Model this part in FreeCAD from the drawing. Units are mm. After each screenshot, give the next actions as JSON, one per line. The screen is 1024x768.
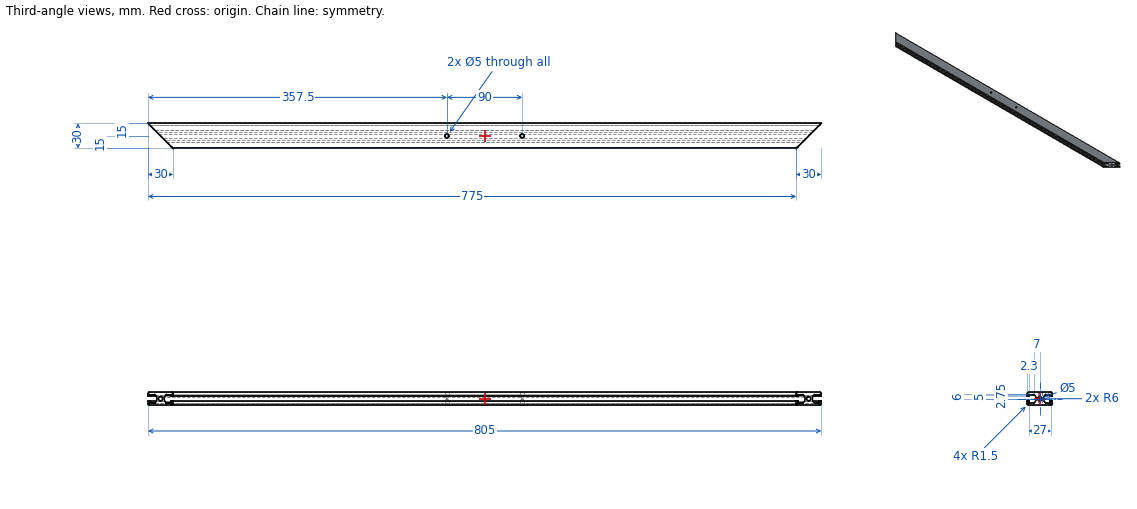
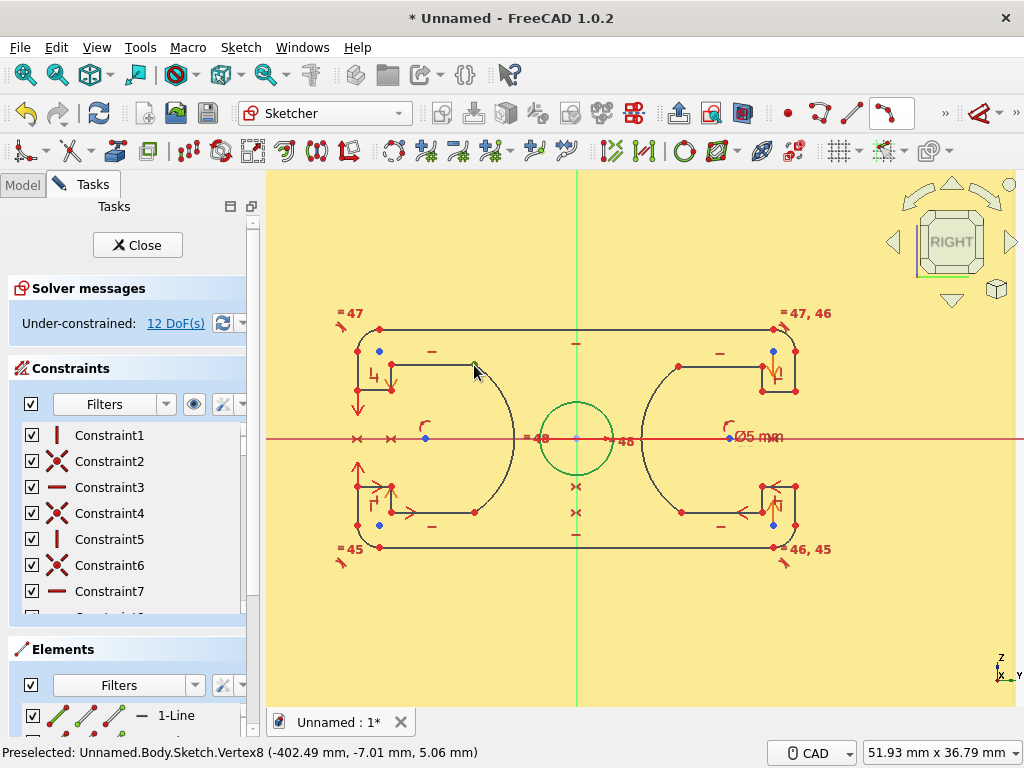
{"action": "left_click", "coordinate": [678, 367]}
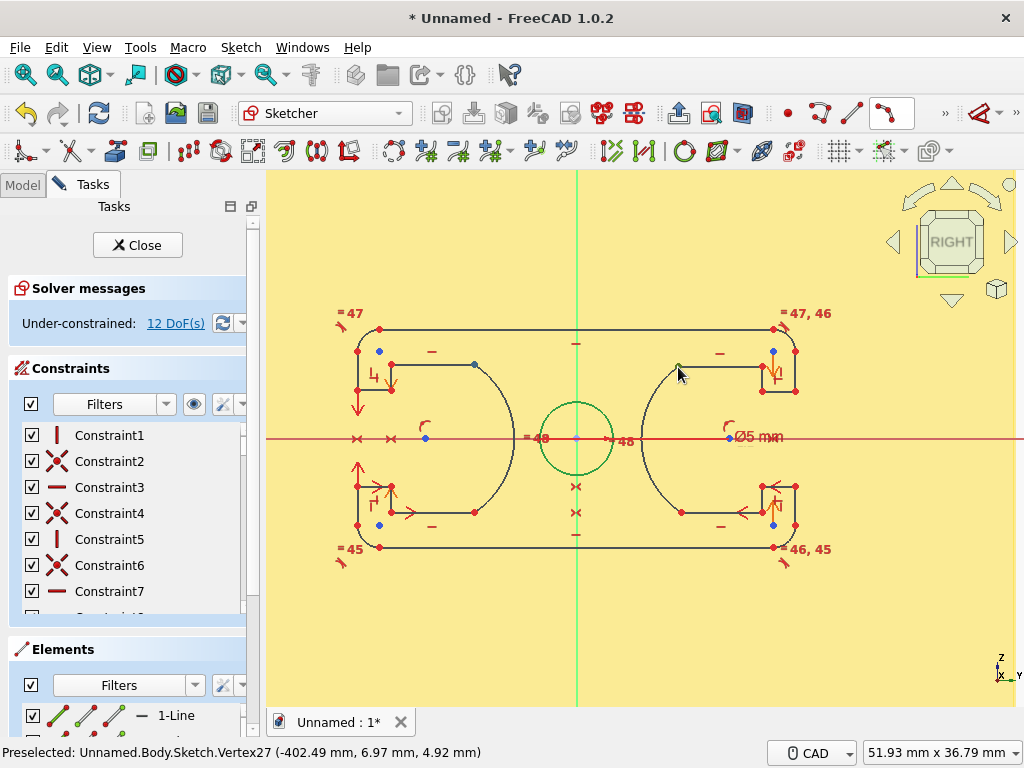
{"action": "left_click", "coordinate": [577, 645]}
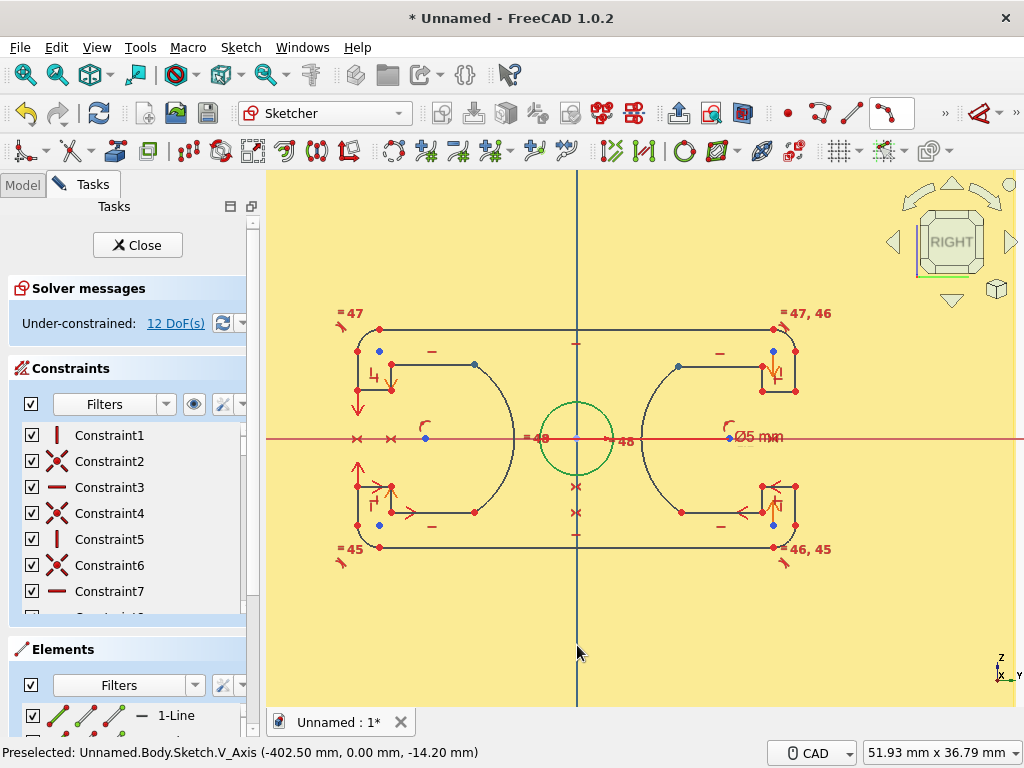
{"action": "key", "text": "s"}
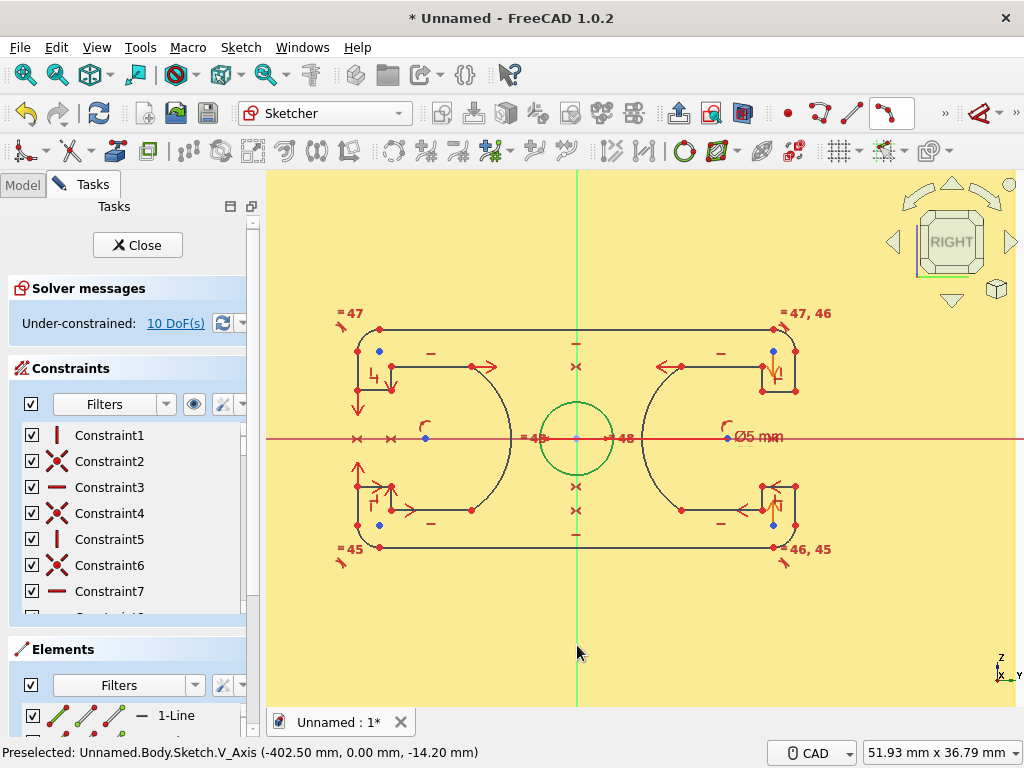
{"action": "left_click", "coordinate": [391, 390]}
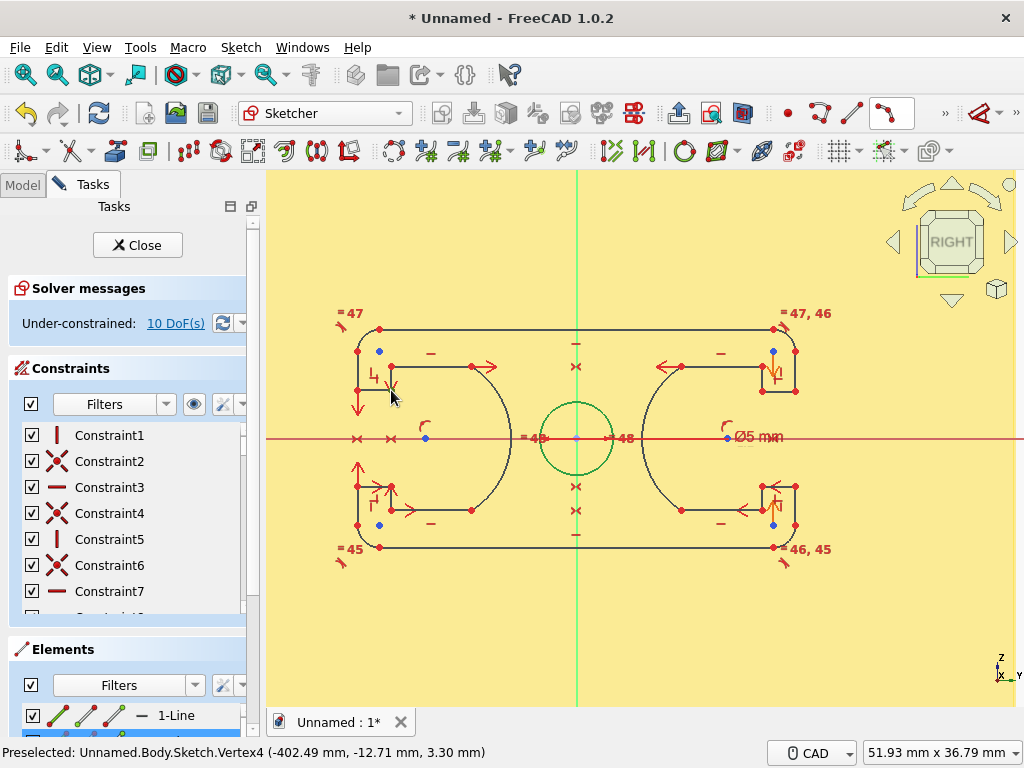
{"action": "left_click", "coordinate": [762, 392]}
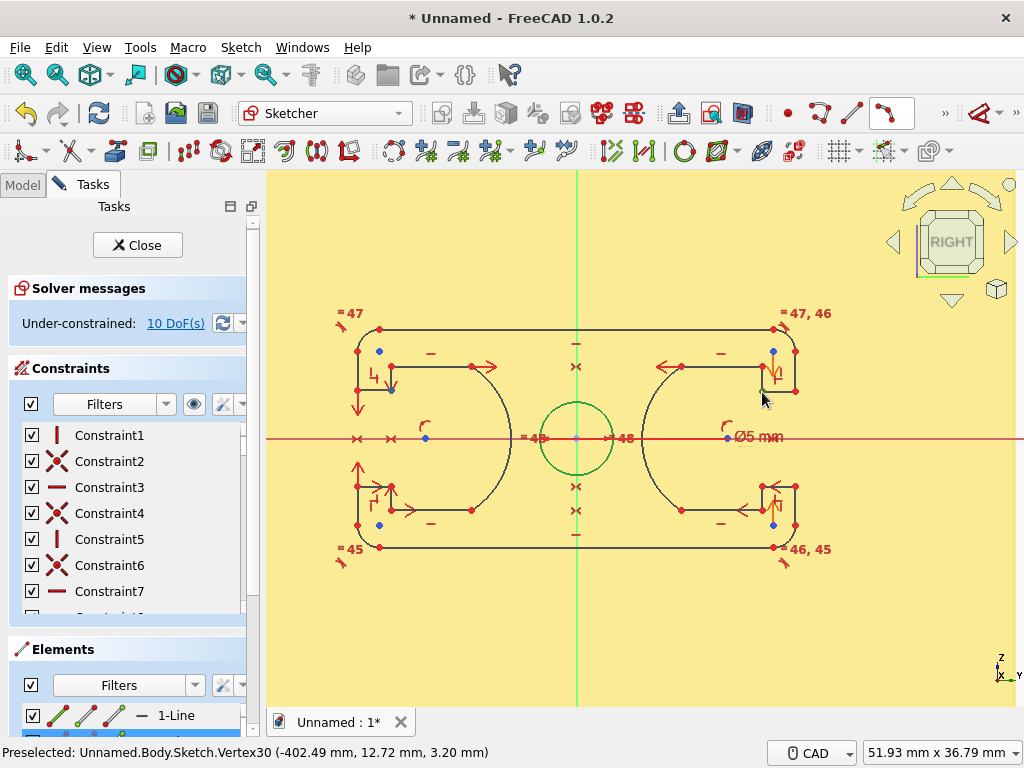
{"action": "left_click", "coordinate": [577, 645]}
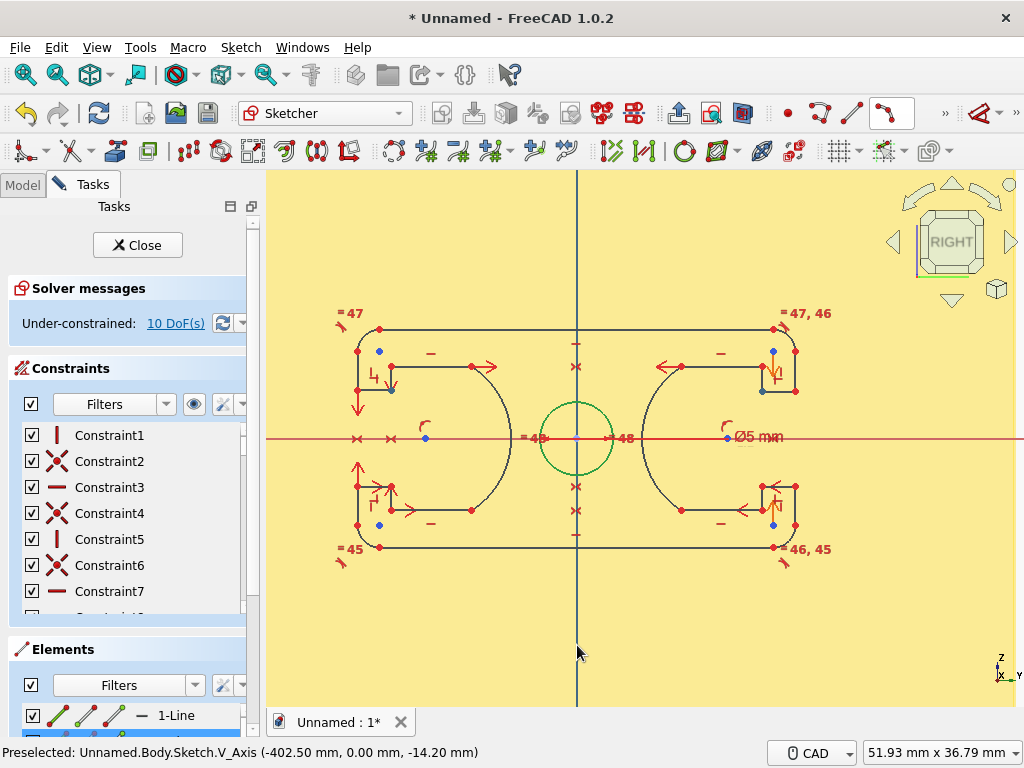
{"action": "key", "text": "s"}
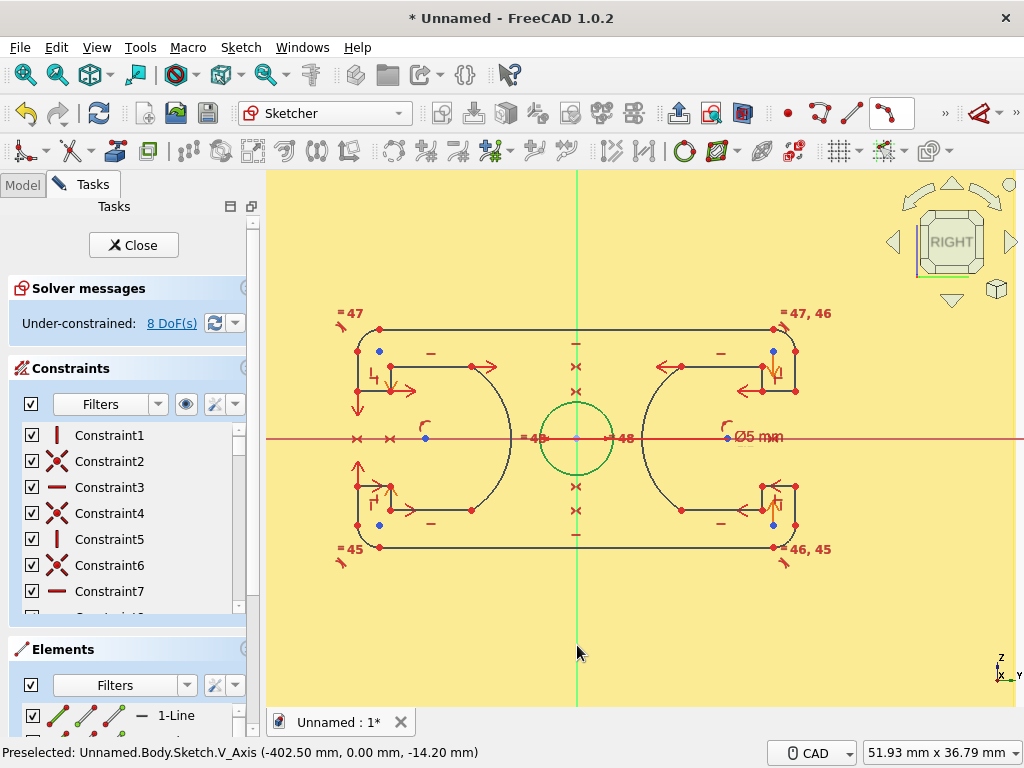
{"action": "left_click", "coordinate": [504, 472]}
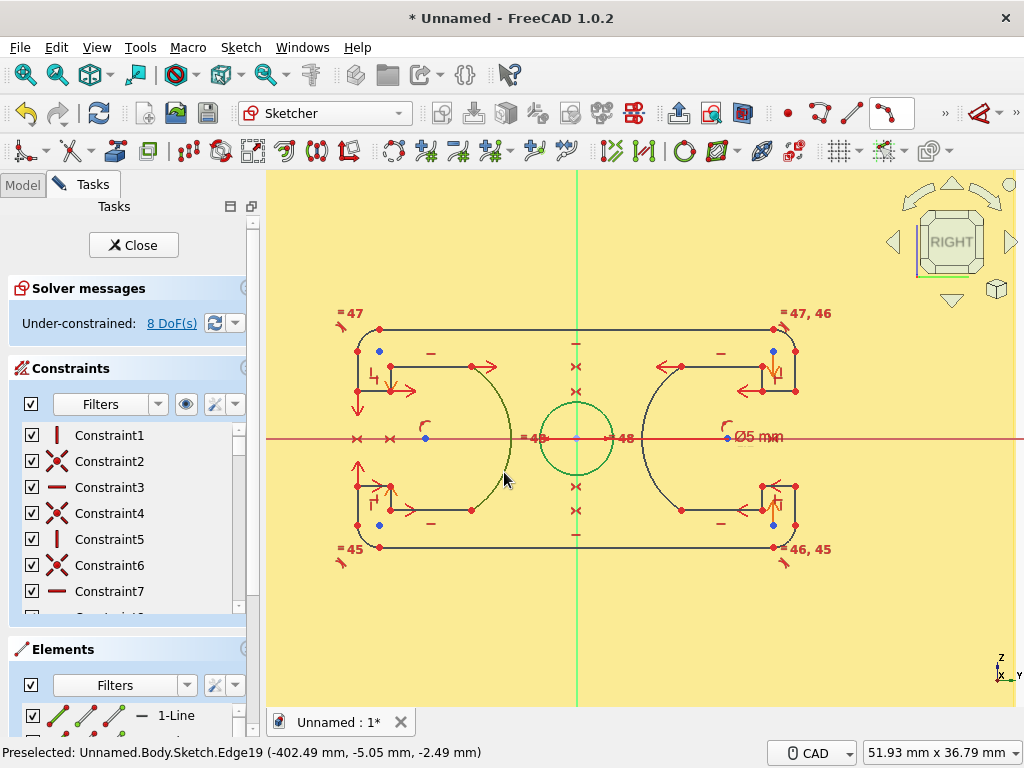
{"action": "key", "text": "k r"}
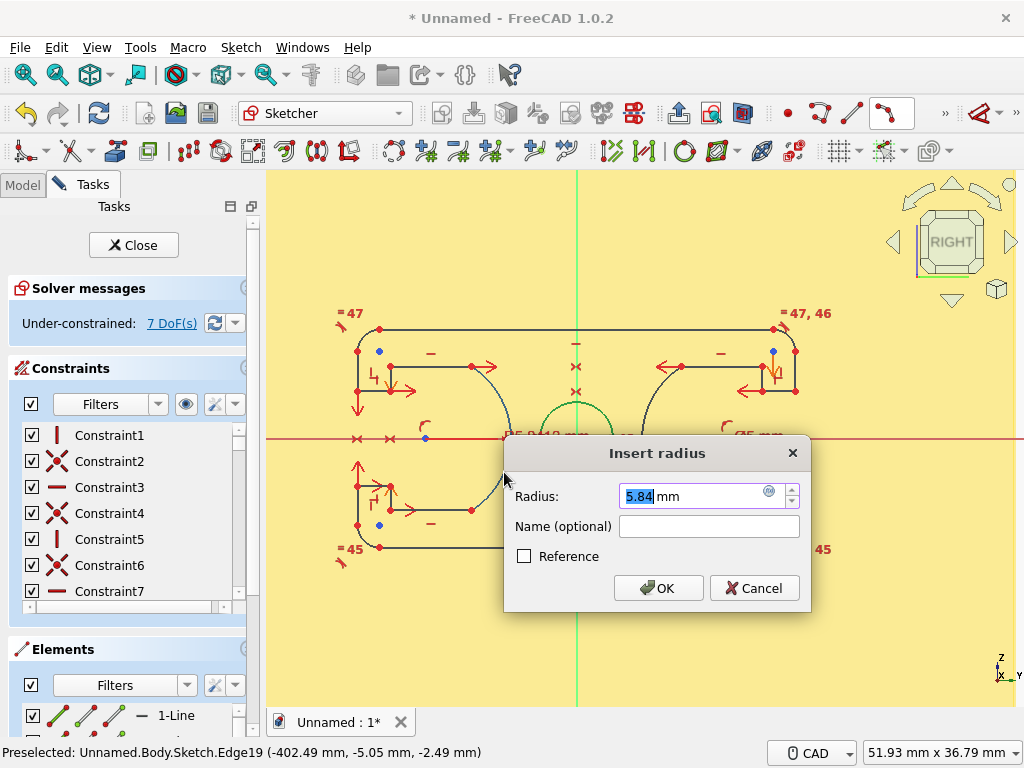
{"action": "type", "text": "6"}
{"action": "key", "text": "Return"}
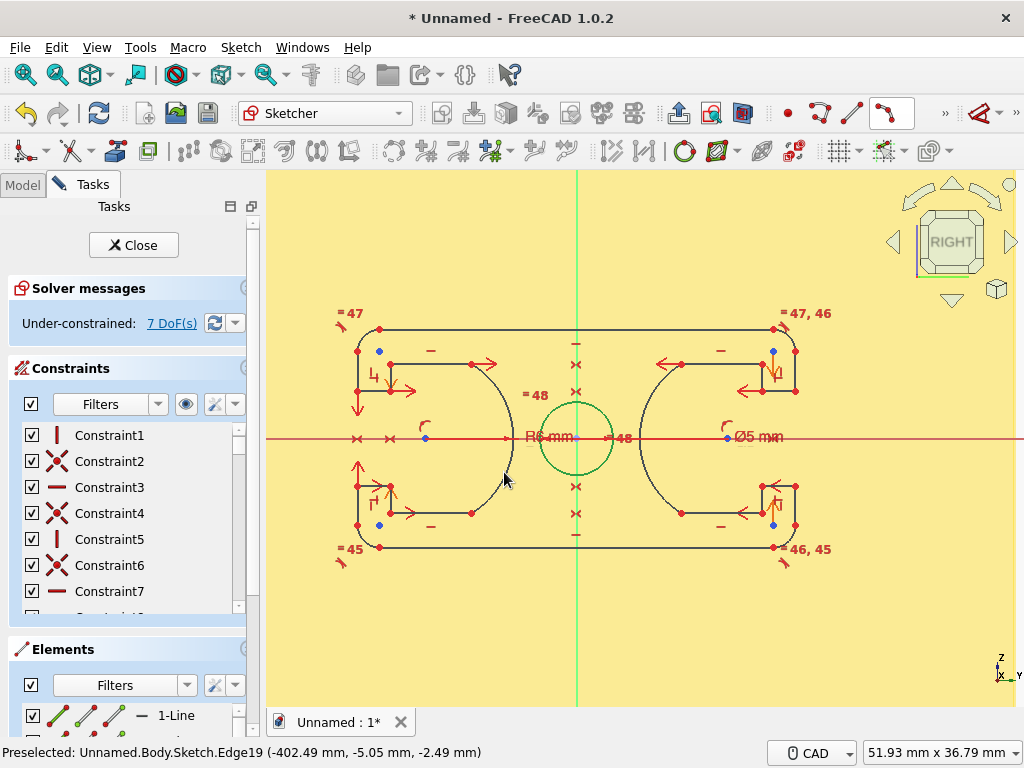
{"action": "scroll", "coordinate": [360, 536], "scroll_direction": "up", "scroll_amount": 3}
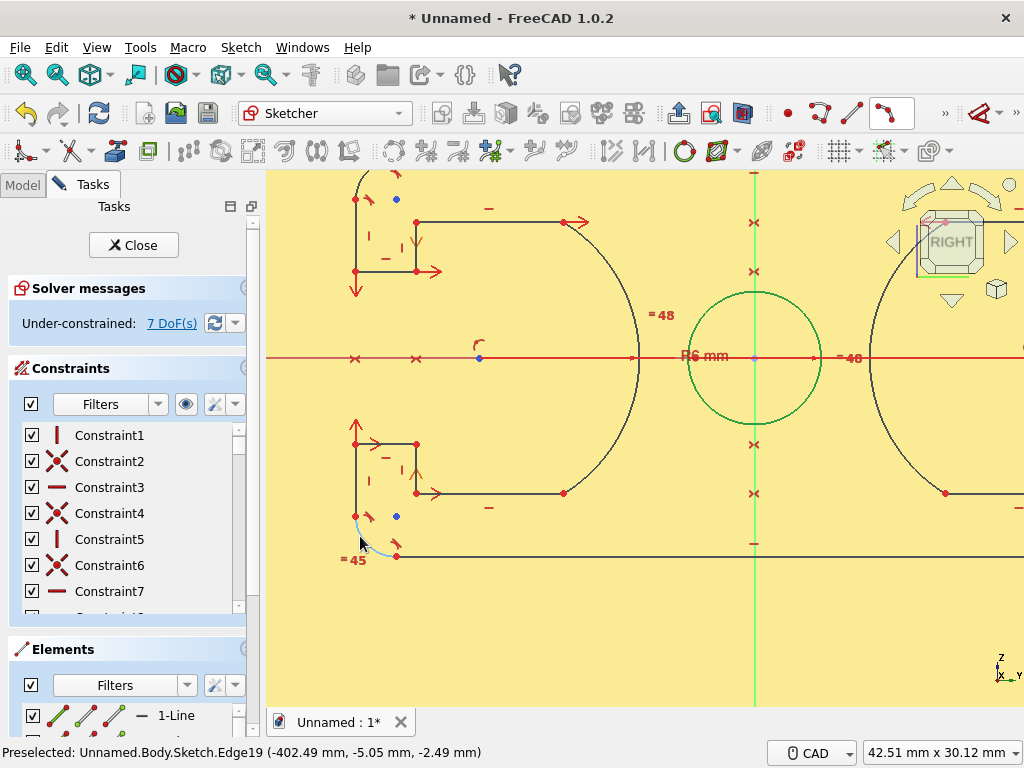
{"action": "left_click", "coordinate": [360, 535]}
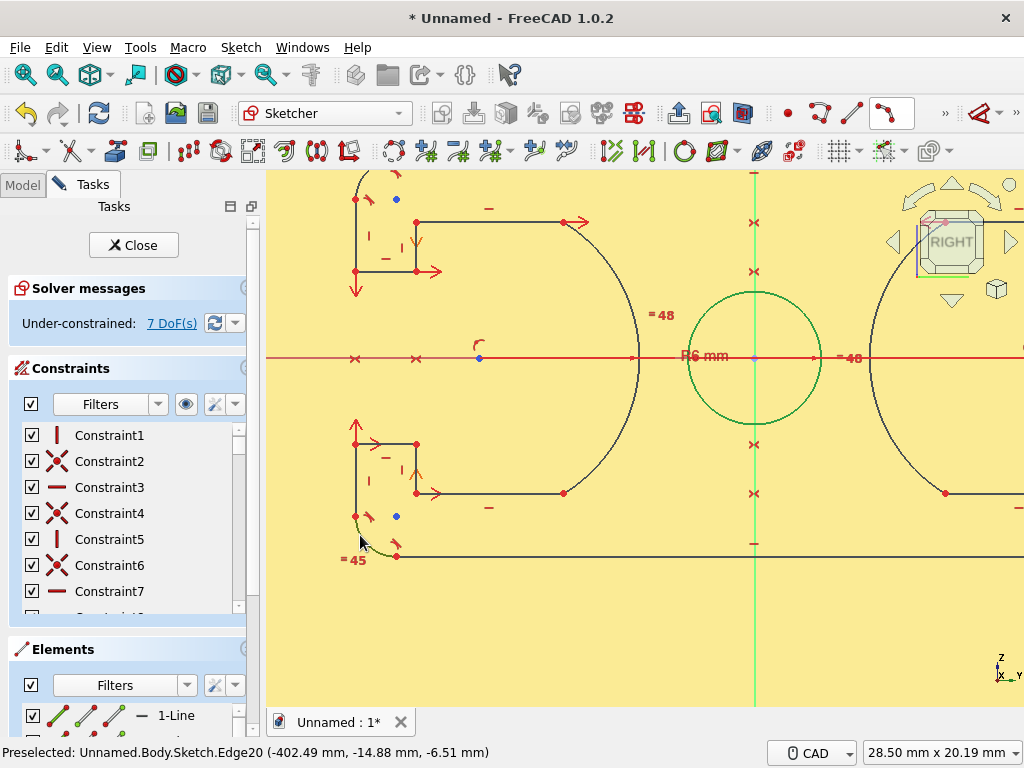
{"action": "left_click", "coordinate": [1002, 114]}